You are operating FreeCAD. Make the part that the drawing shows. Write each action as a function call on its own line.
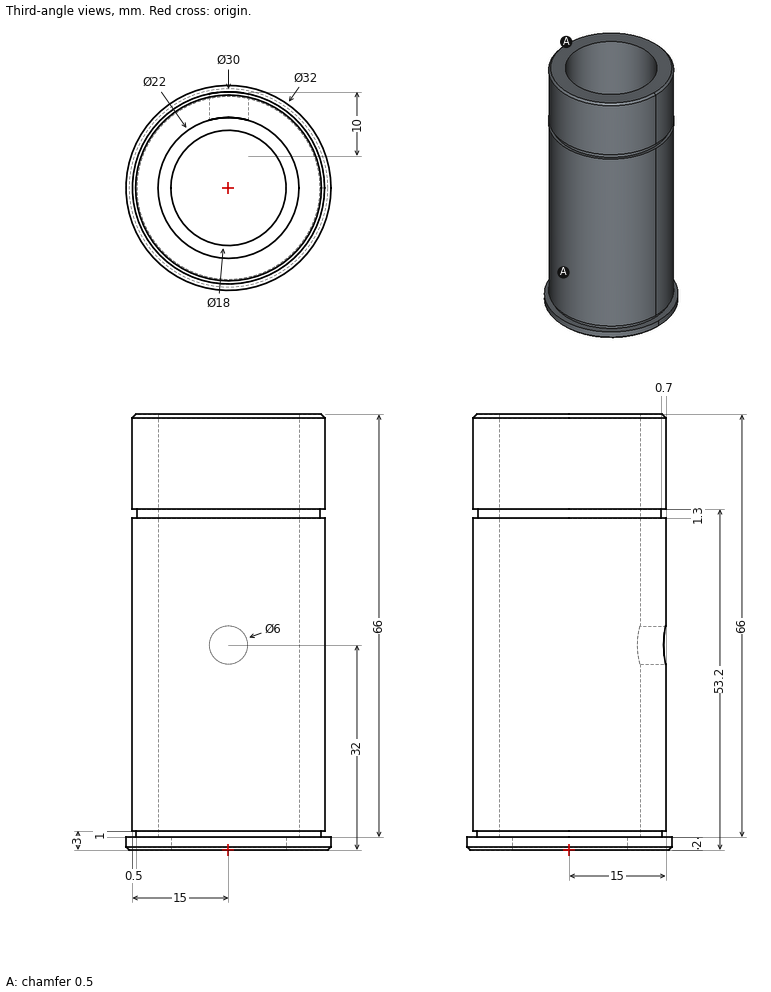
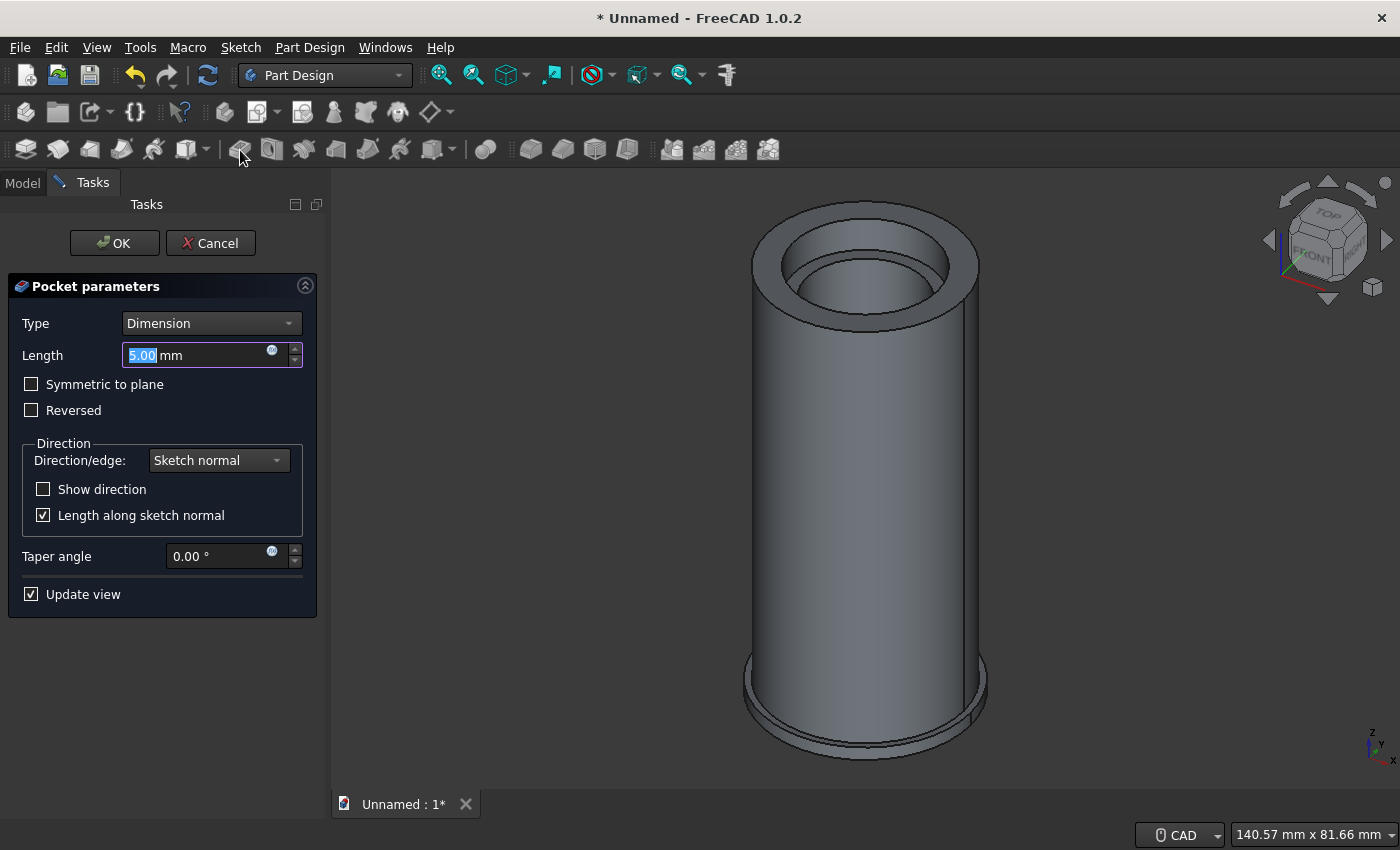
text(66)
key(Tab)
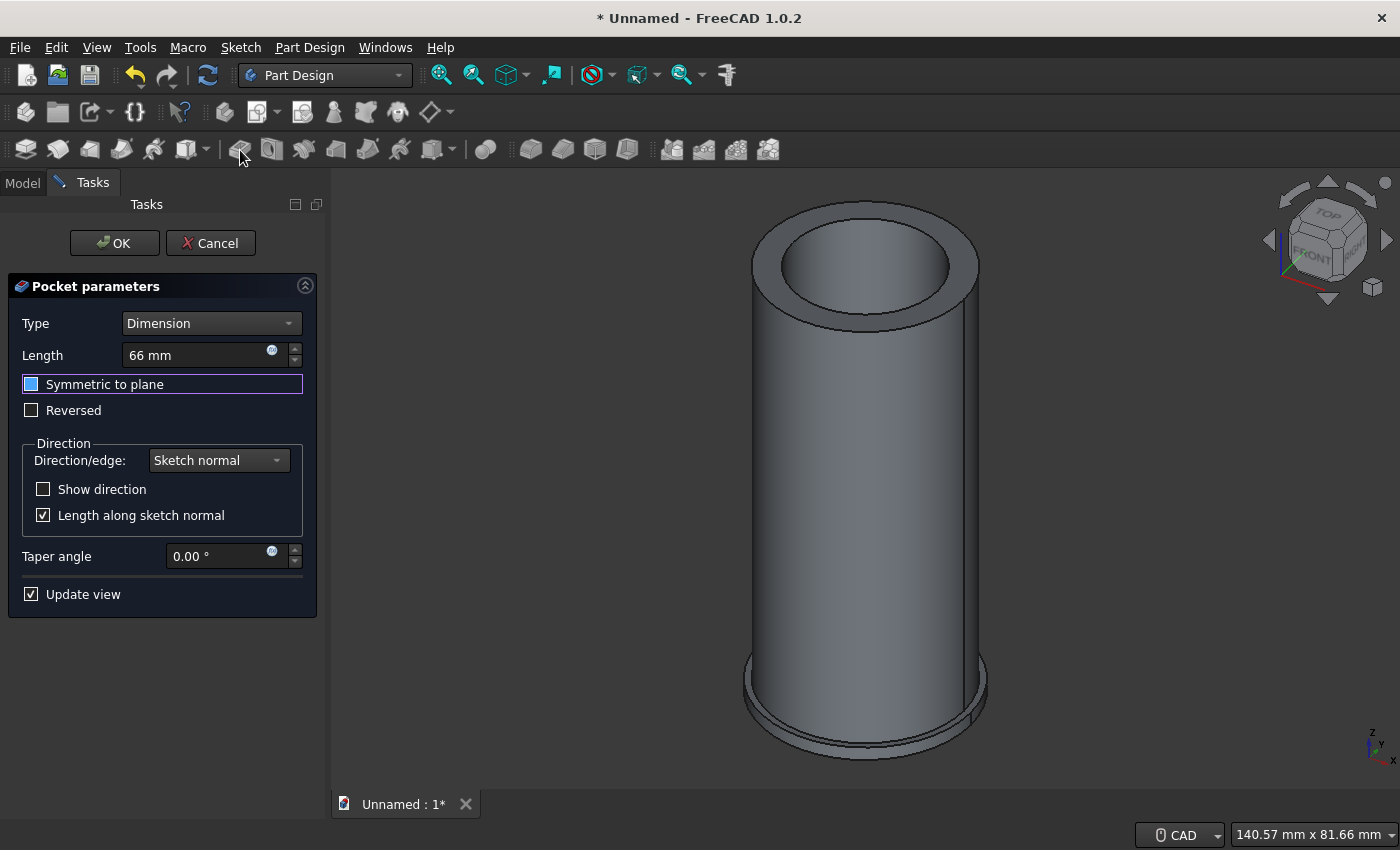
click(115, 243)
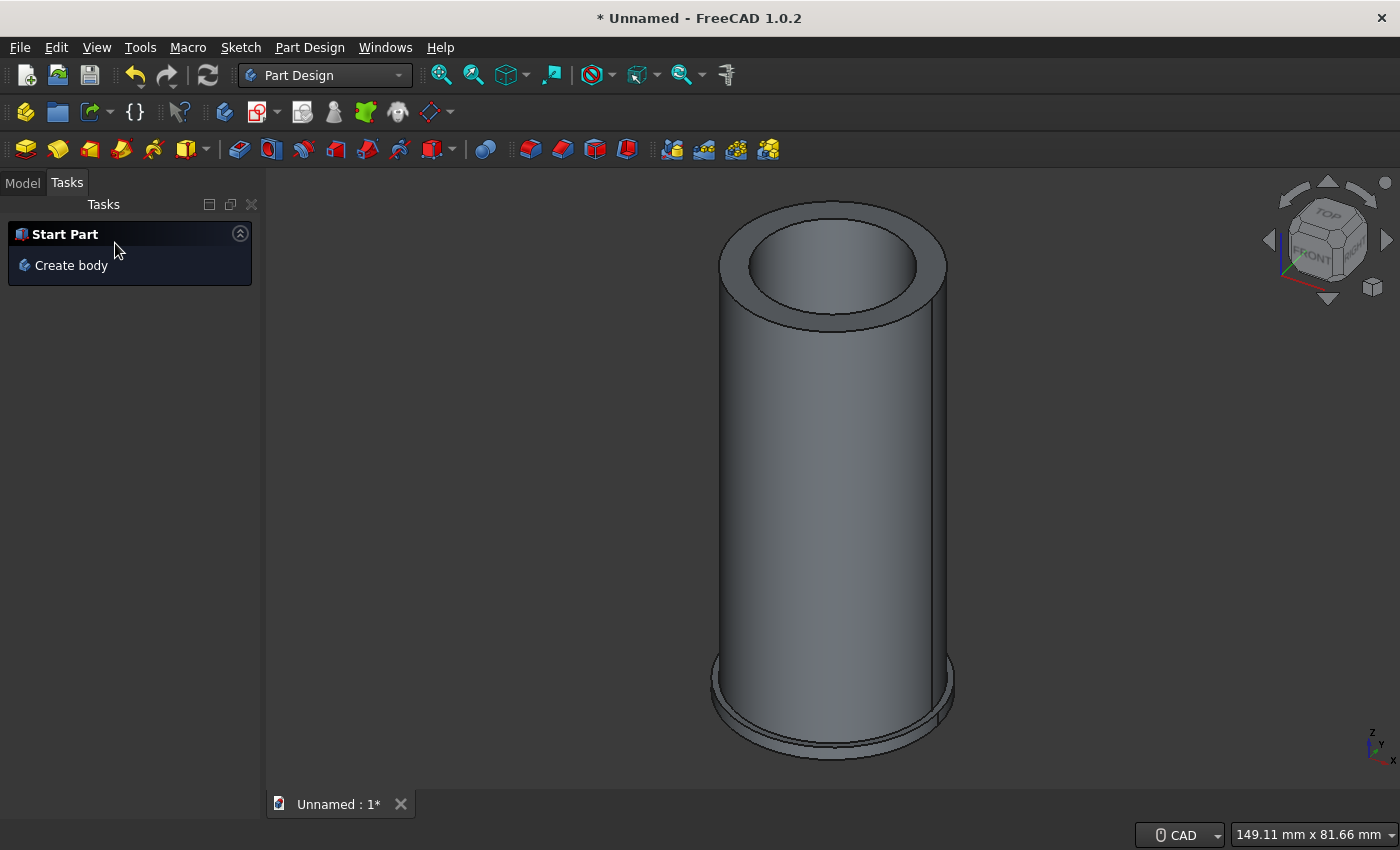
click(23, 182)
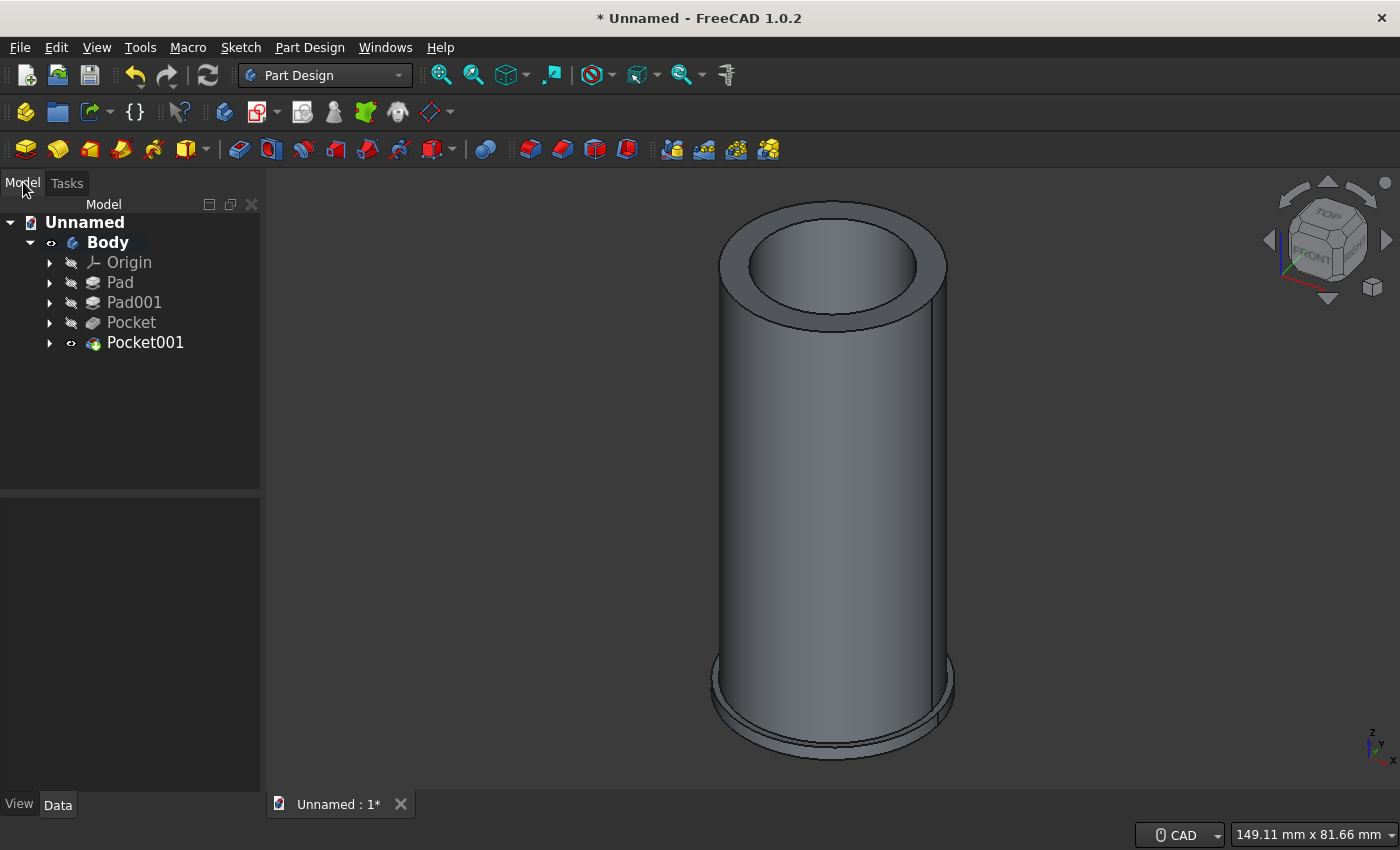
click(50, 263)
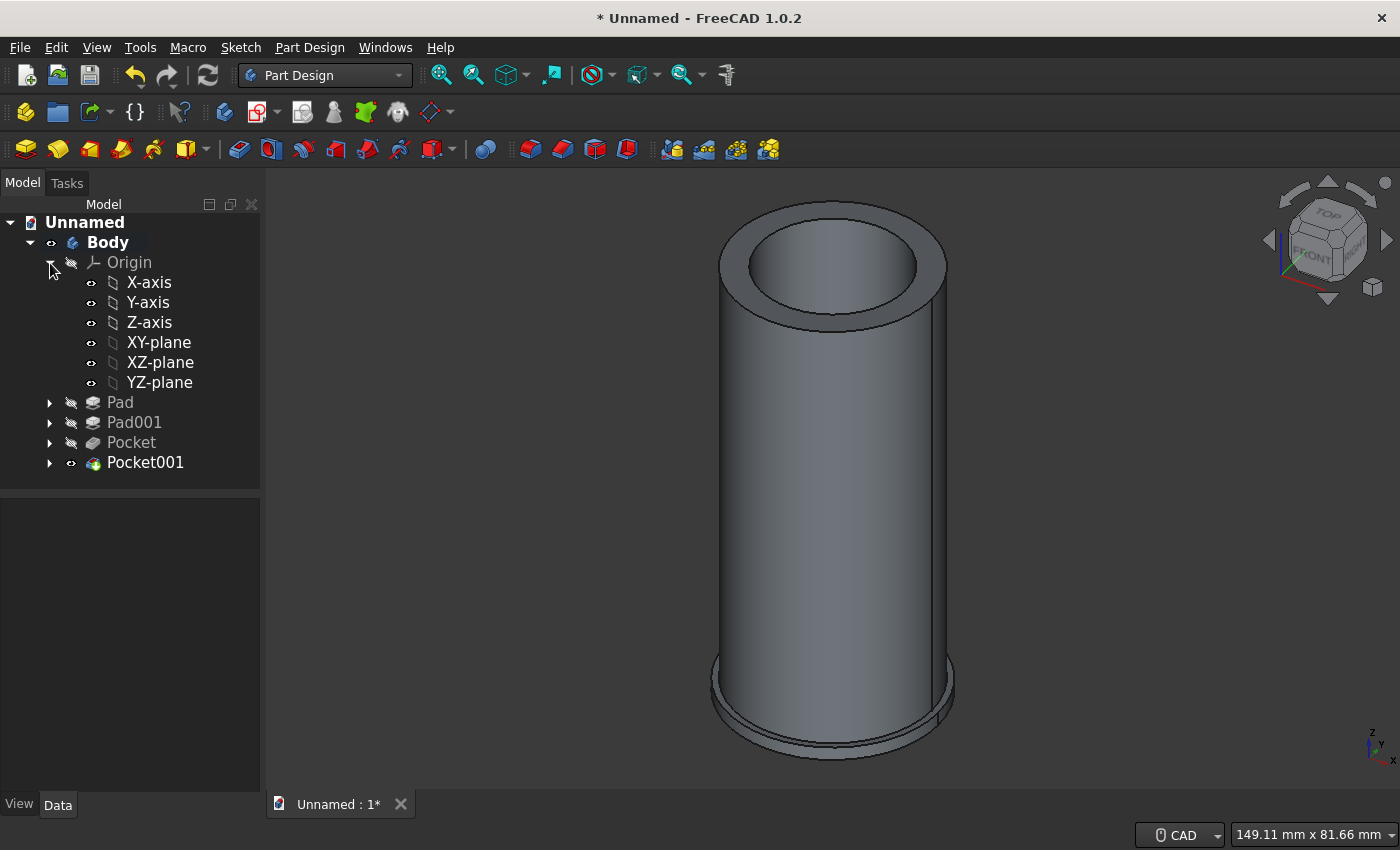
click(136, 363)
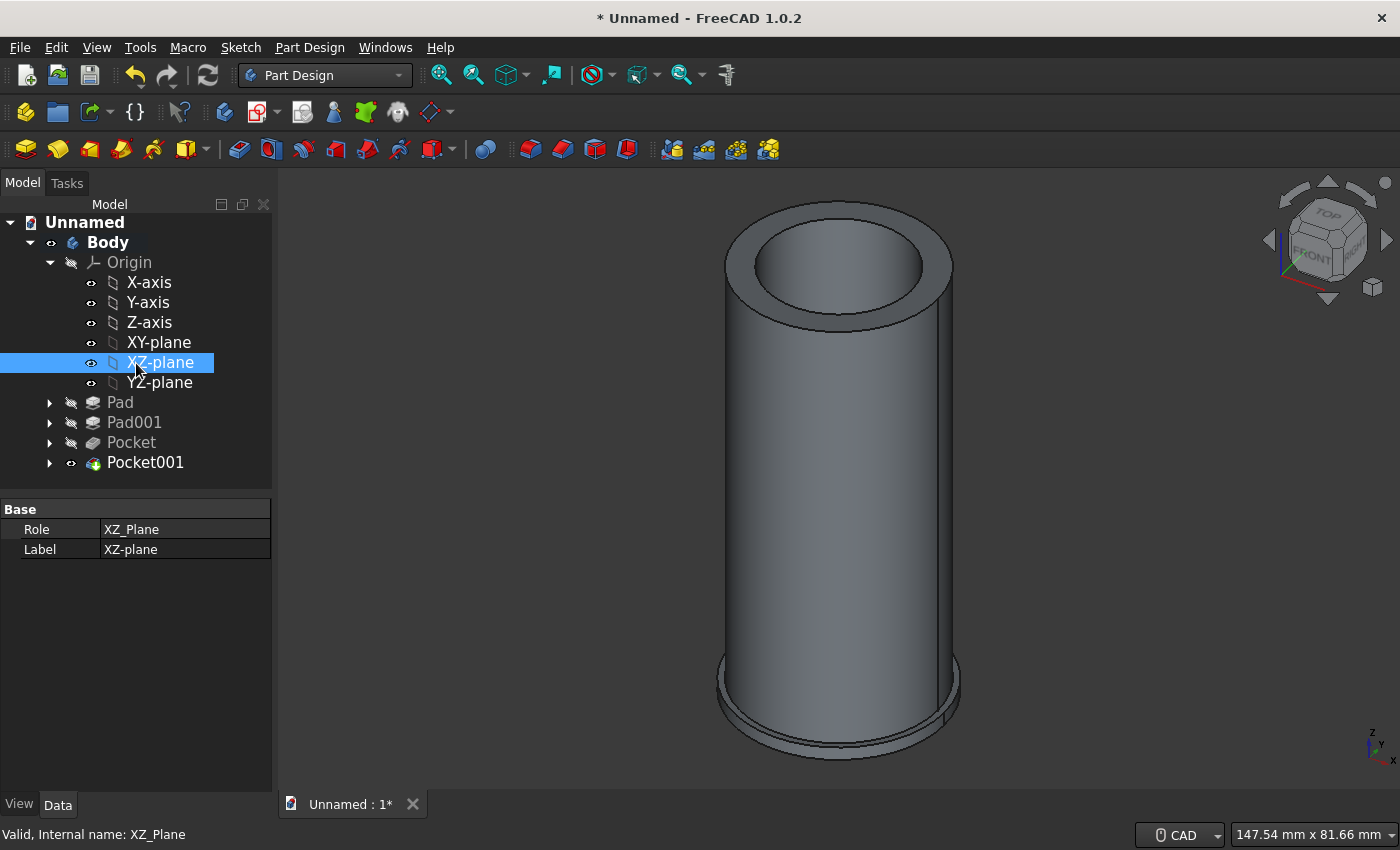
click(430, 112)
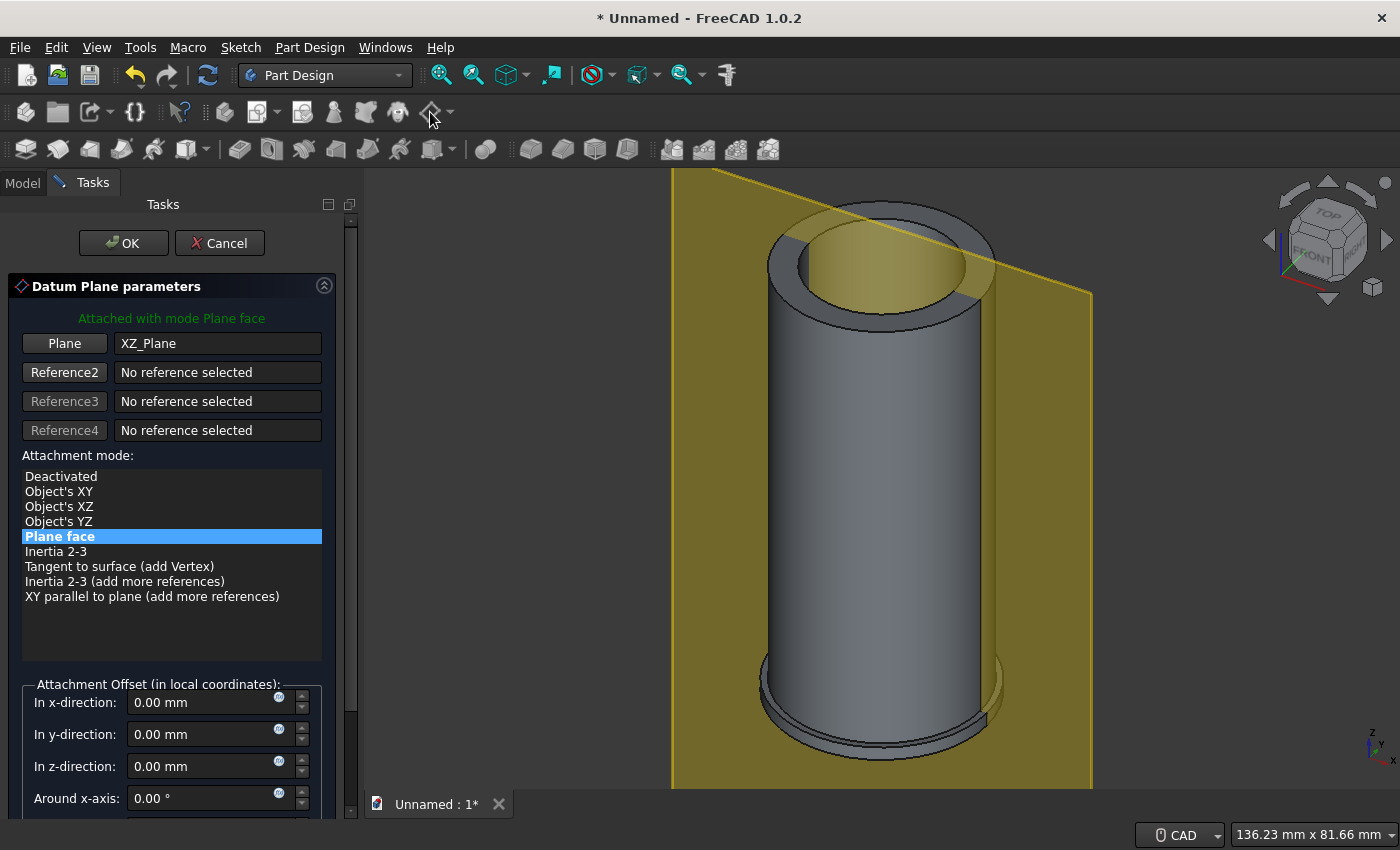
triple_click(210, 766)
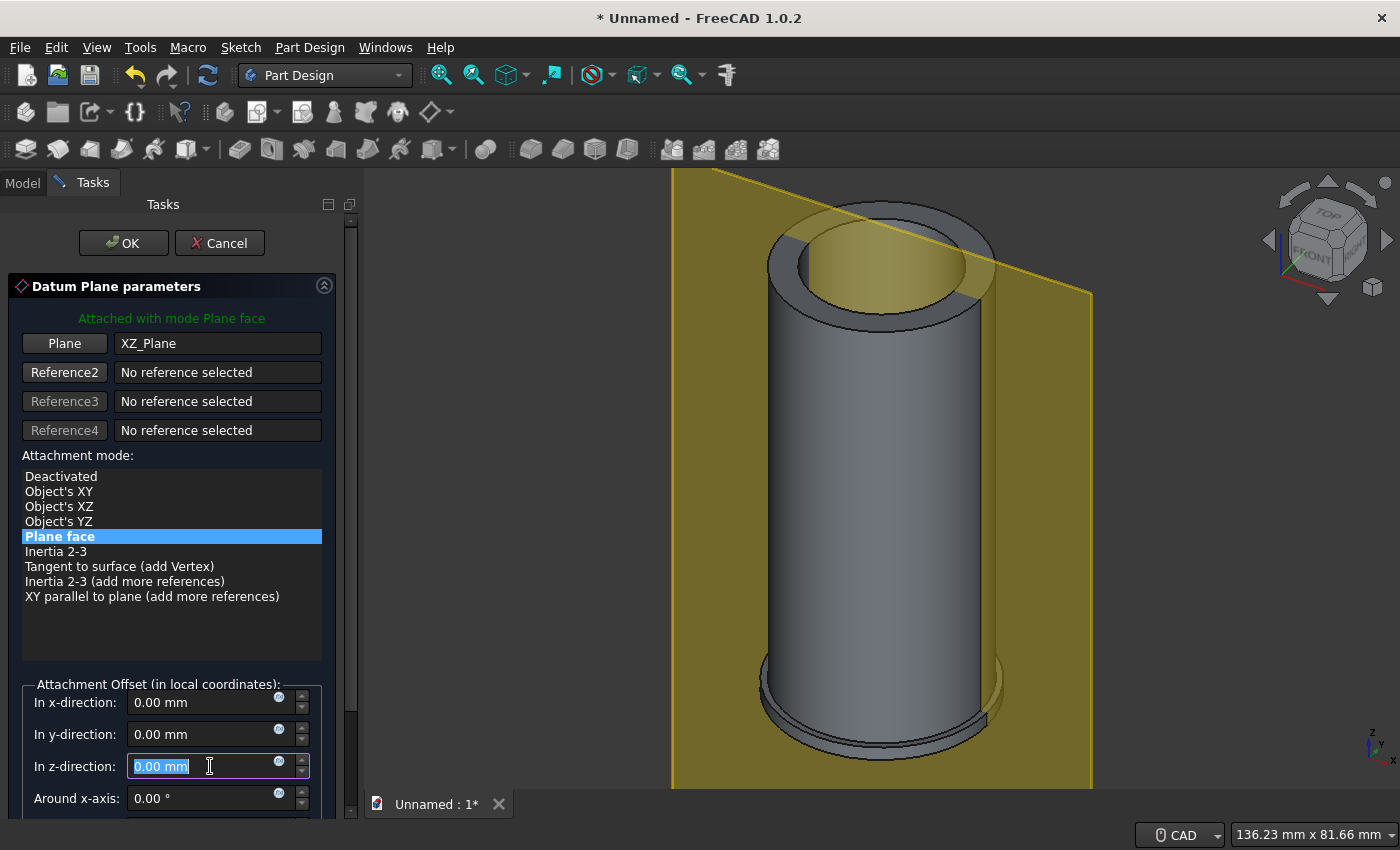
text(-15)
key(Tab)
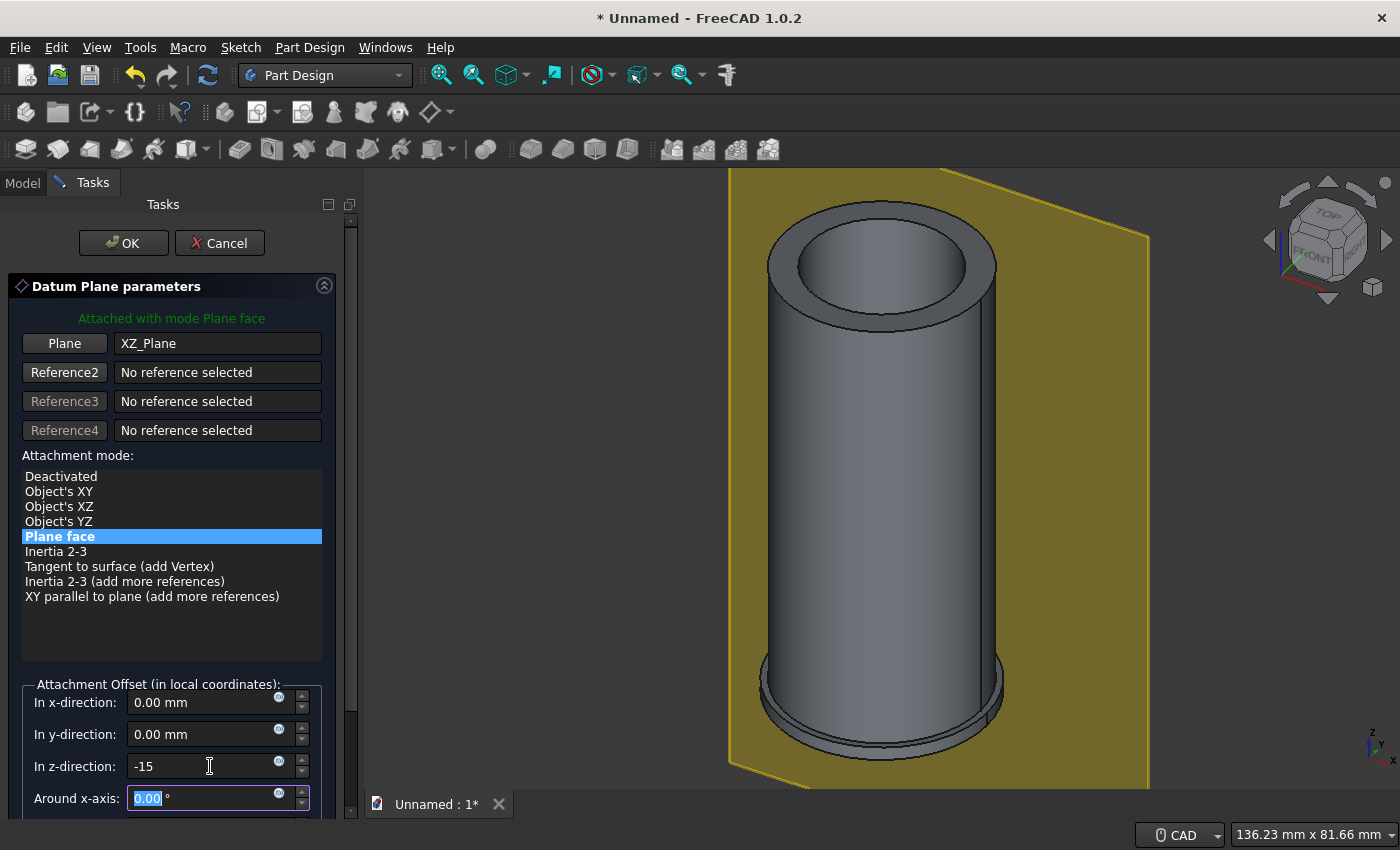
click(124, 243)